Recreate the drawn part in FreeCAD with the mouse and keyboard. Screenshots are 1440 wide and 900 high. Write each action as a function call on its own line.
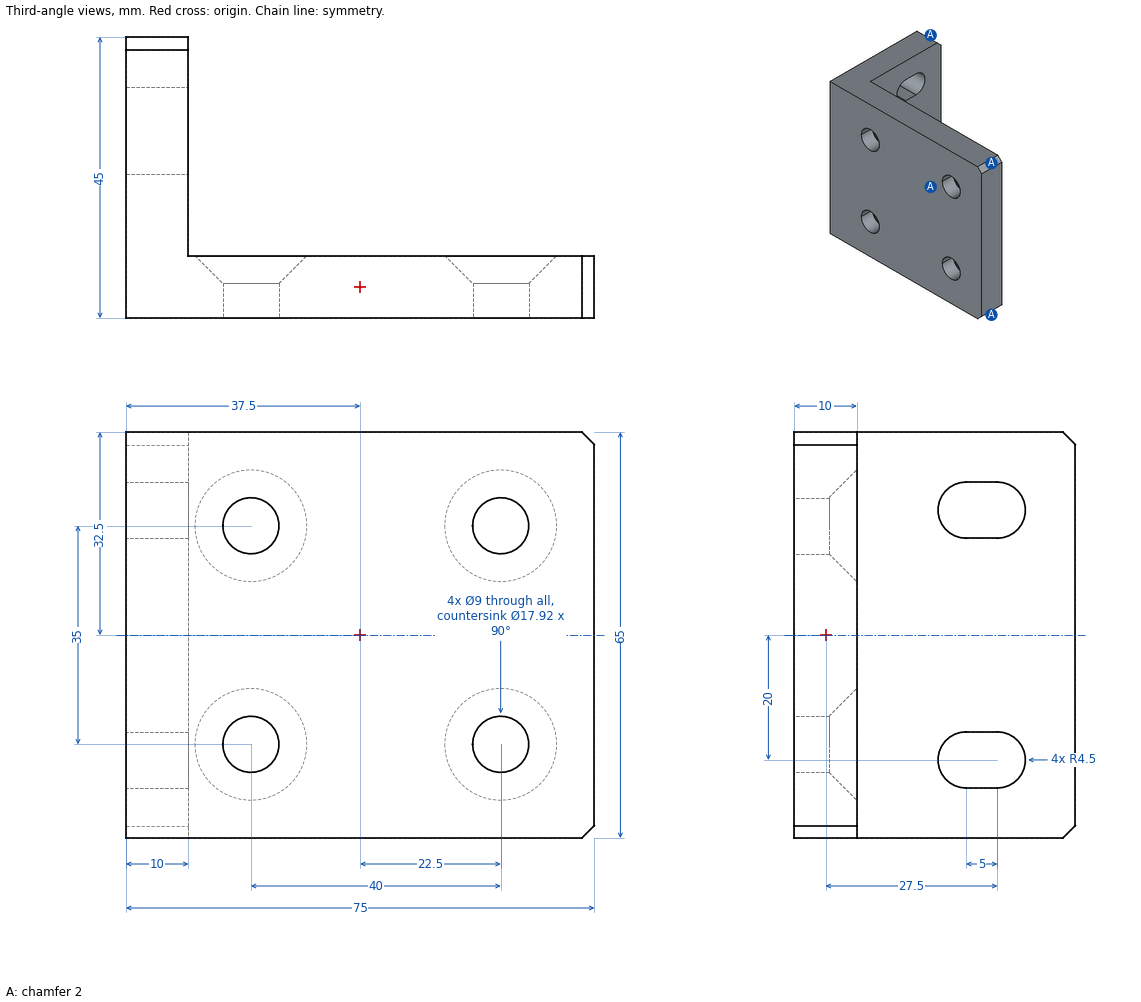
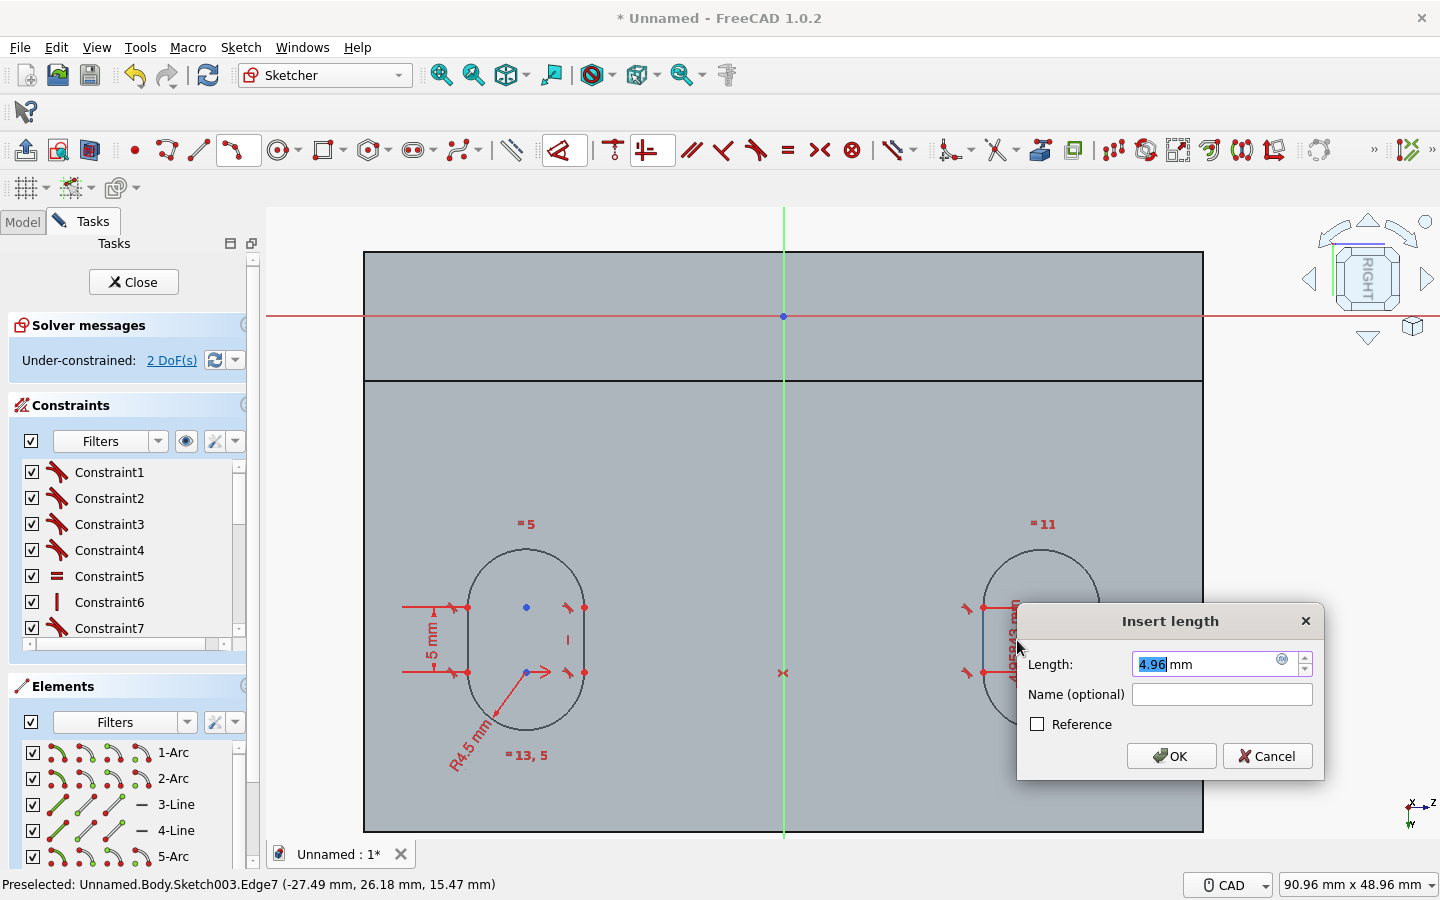
text(5)
key(Return)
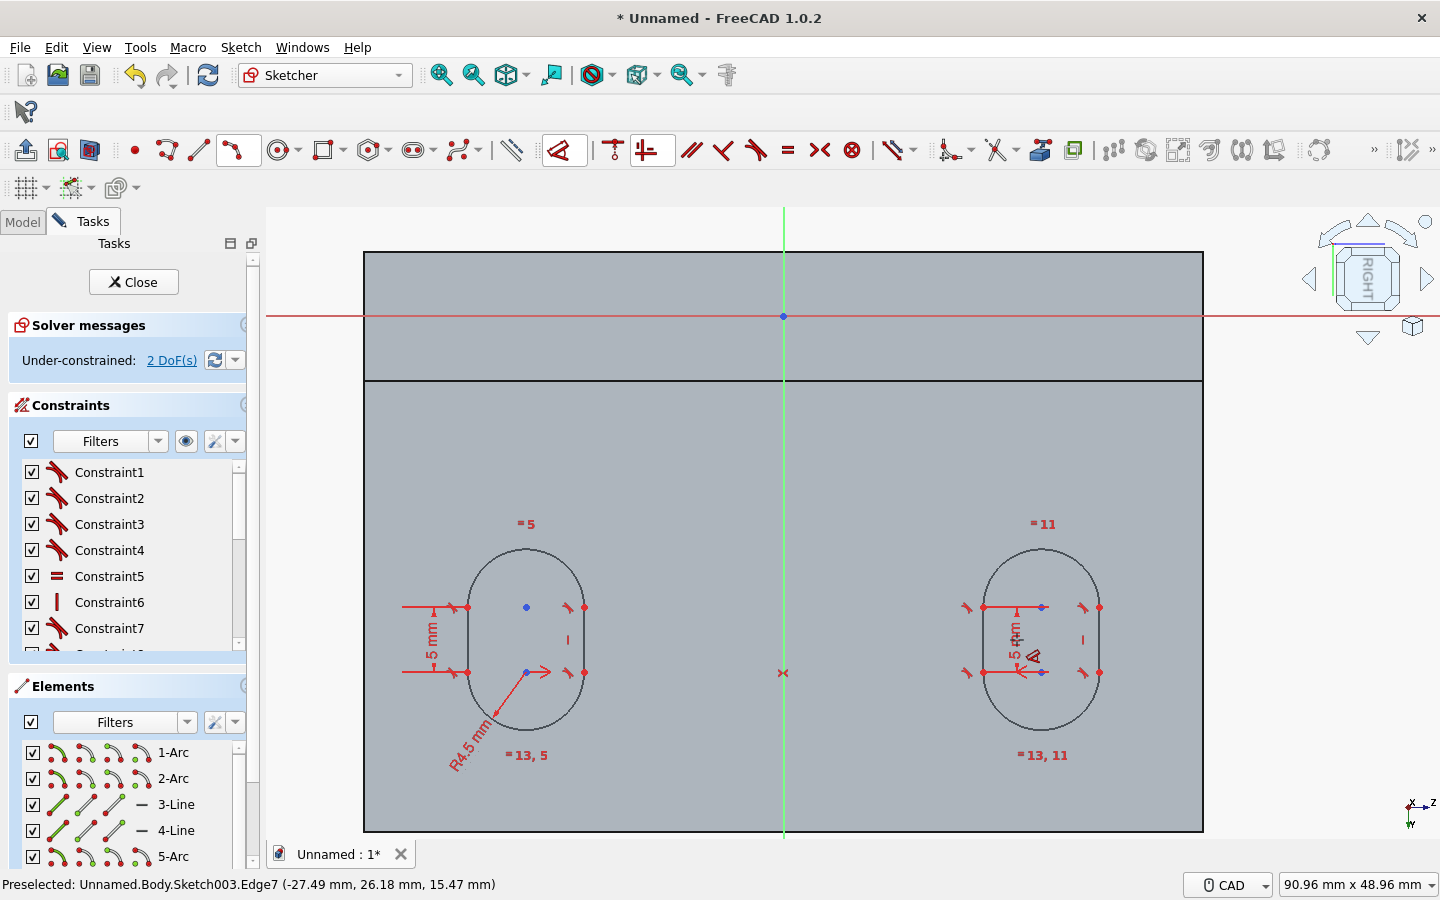
click(526, 672)
click(655, 282)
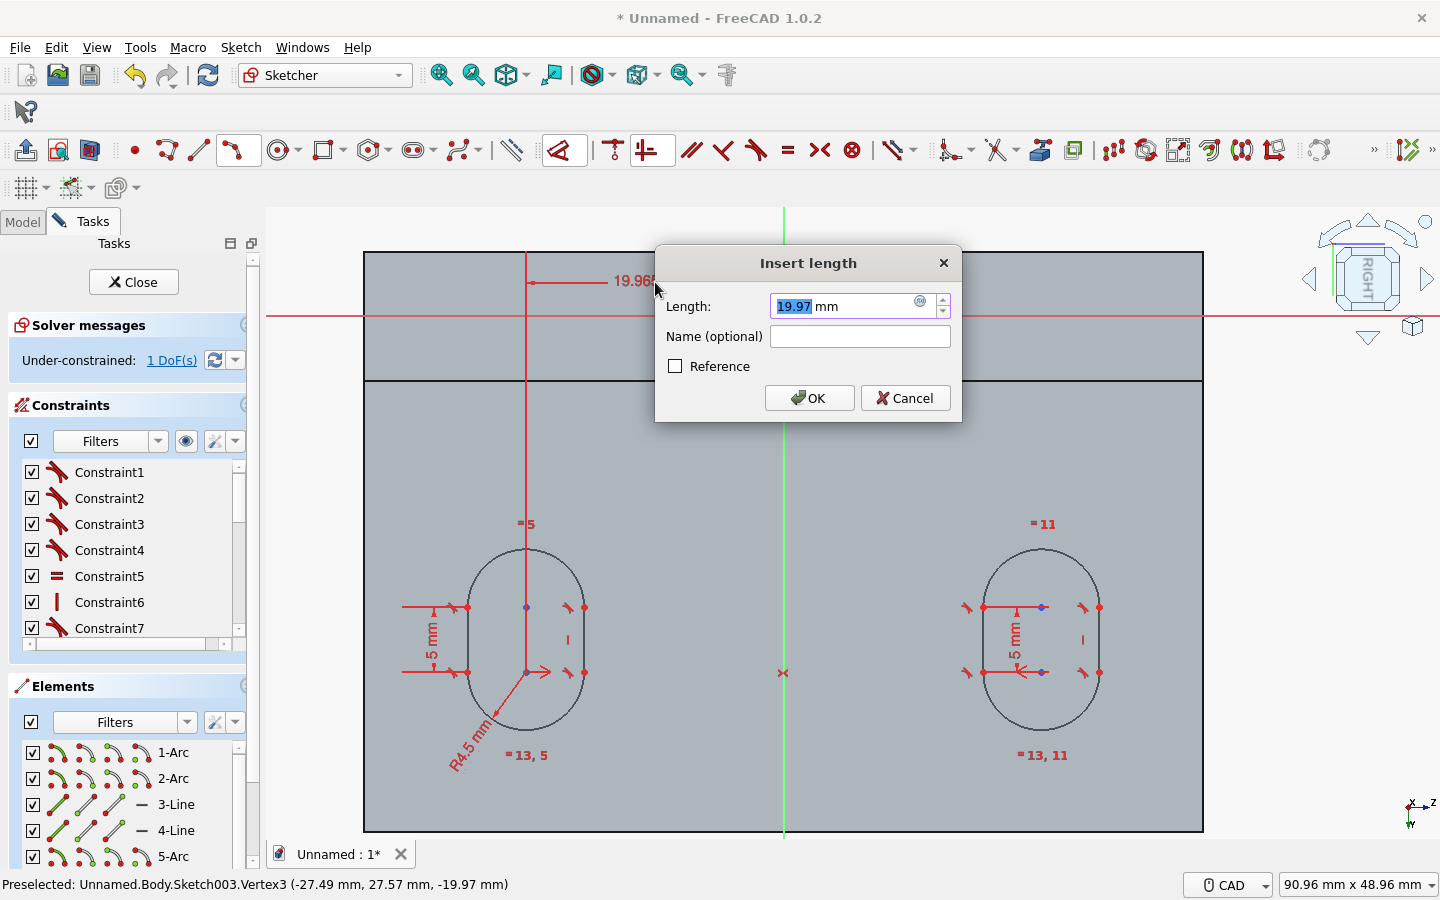
text(20)
key(Return)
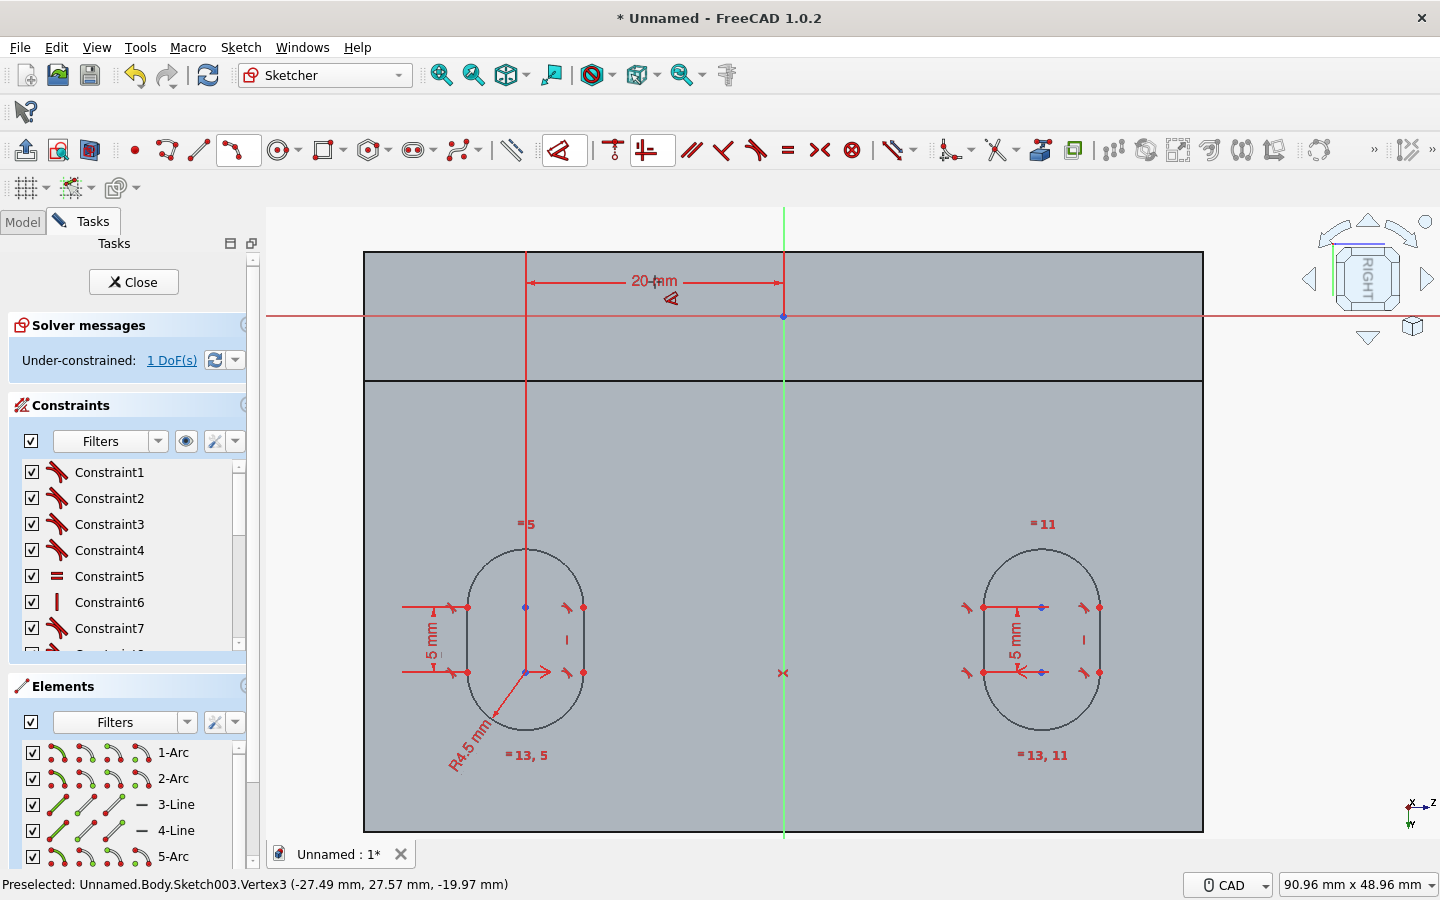
click(467, 672)
click(433, 494)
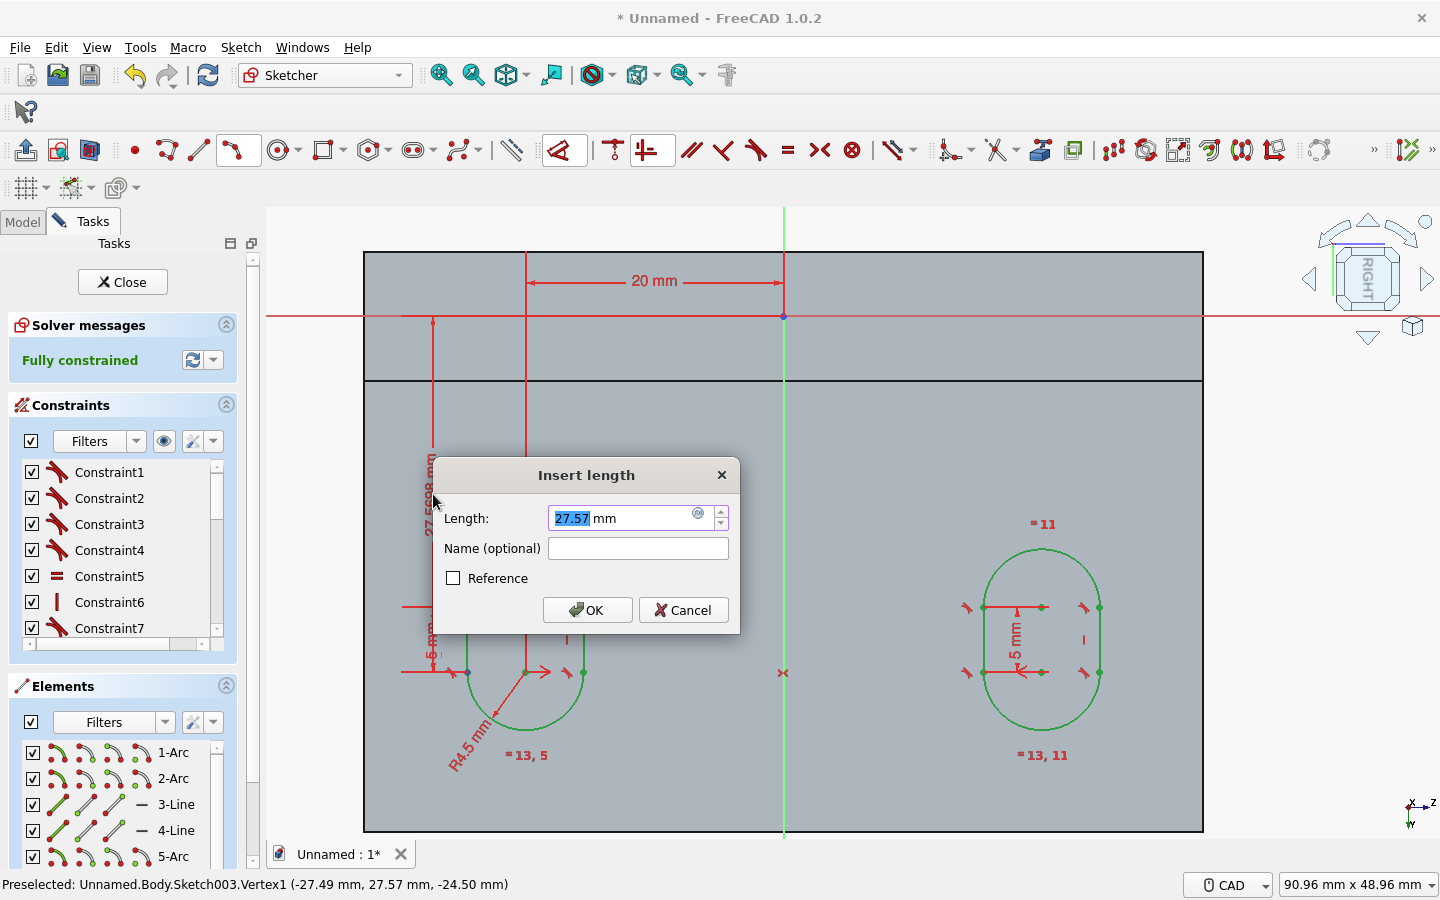
text(27.5)
key(Return)
key(Escape)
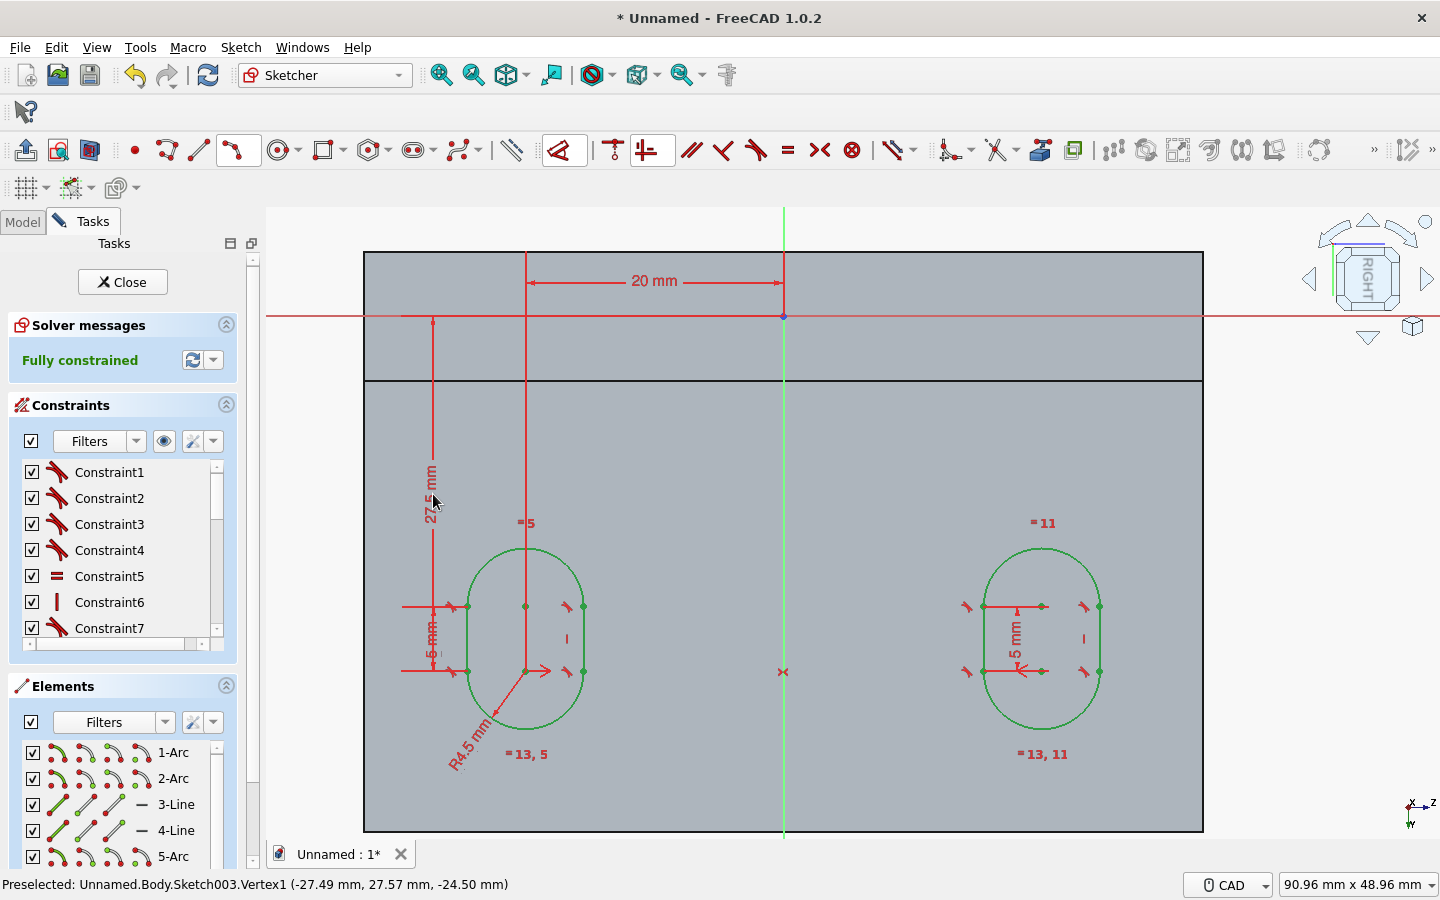
click(123, 282)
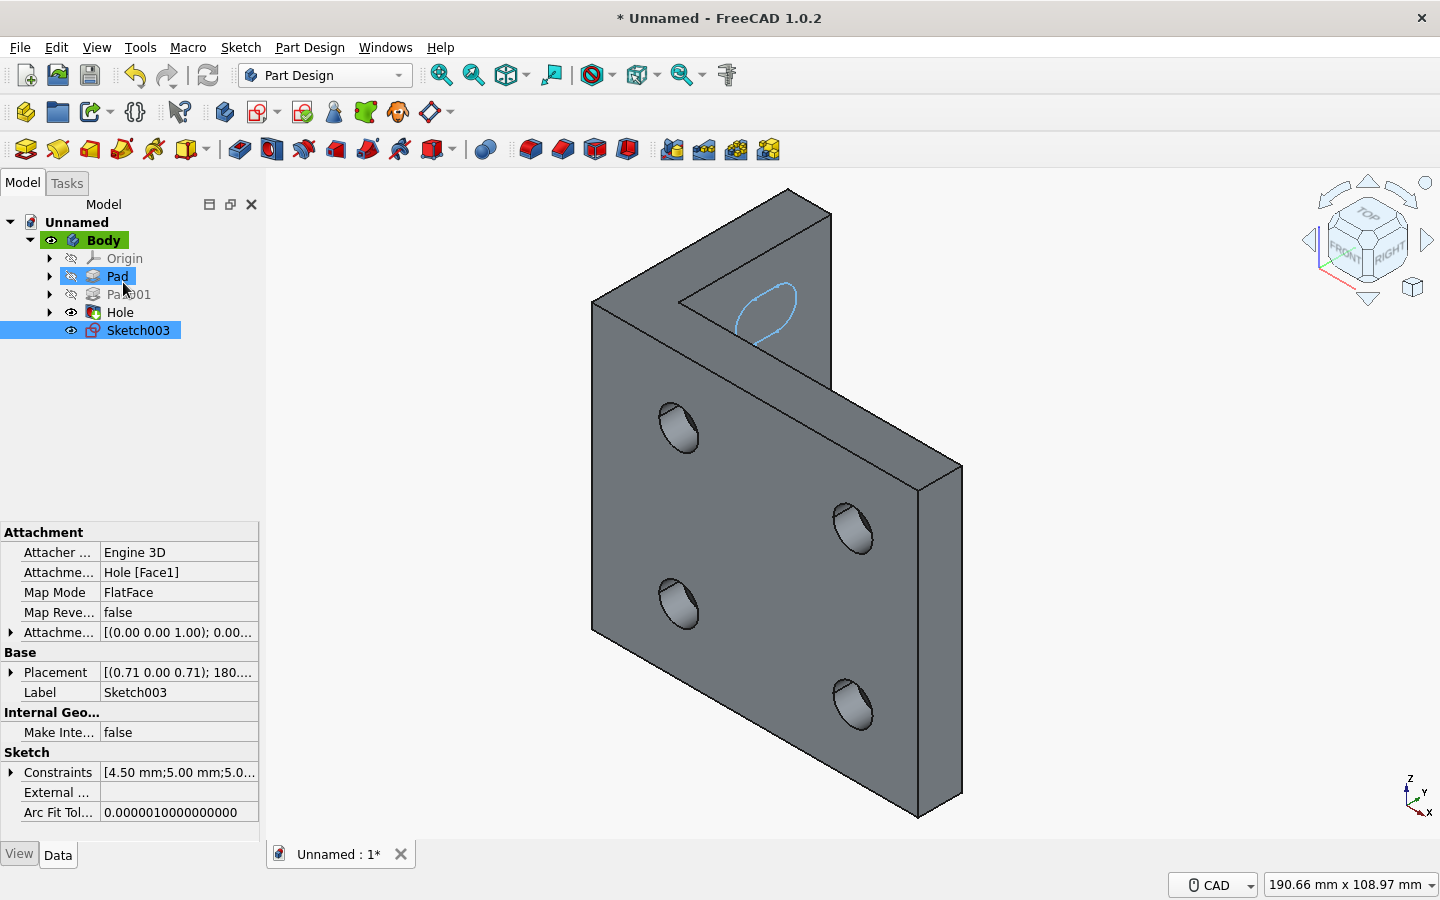
click(240, 150)